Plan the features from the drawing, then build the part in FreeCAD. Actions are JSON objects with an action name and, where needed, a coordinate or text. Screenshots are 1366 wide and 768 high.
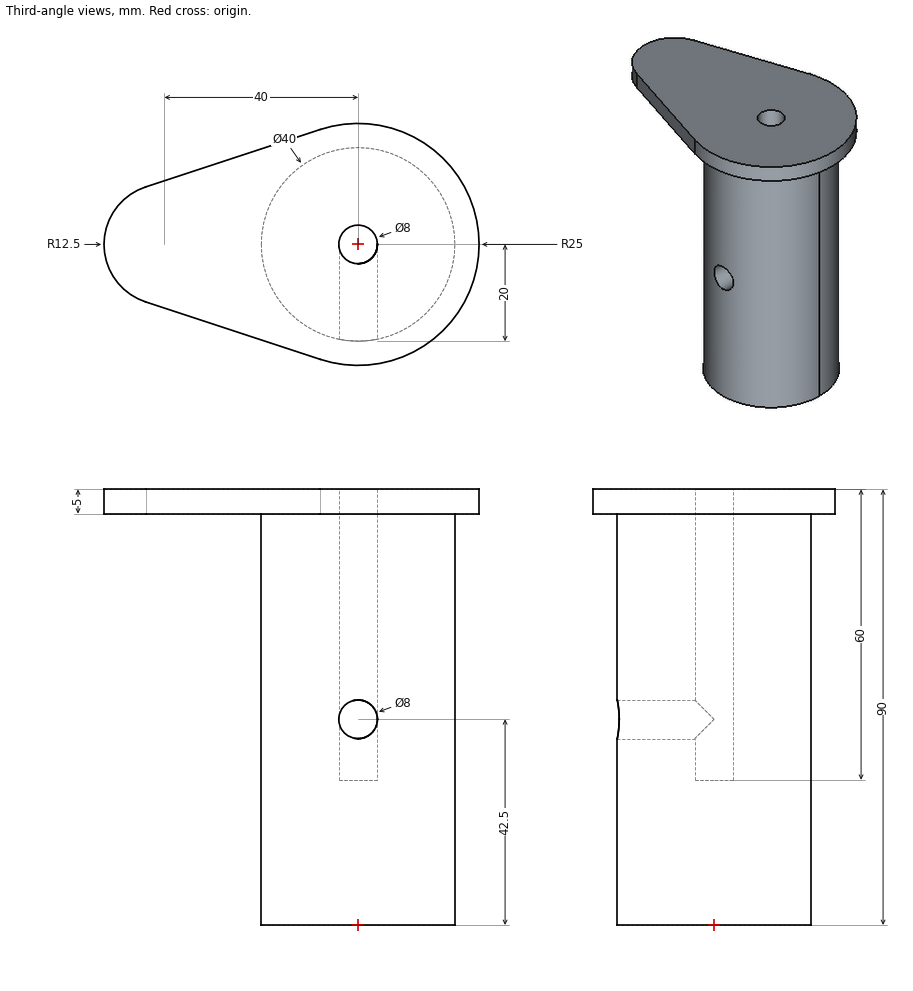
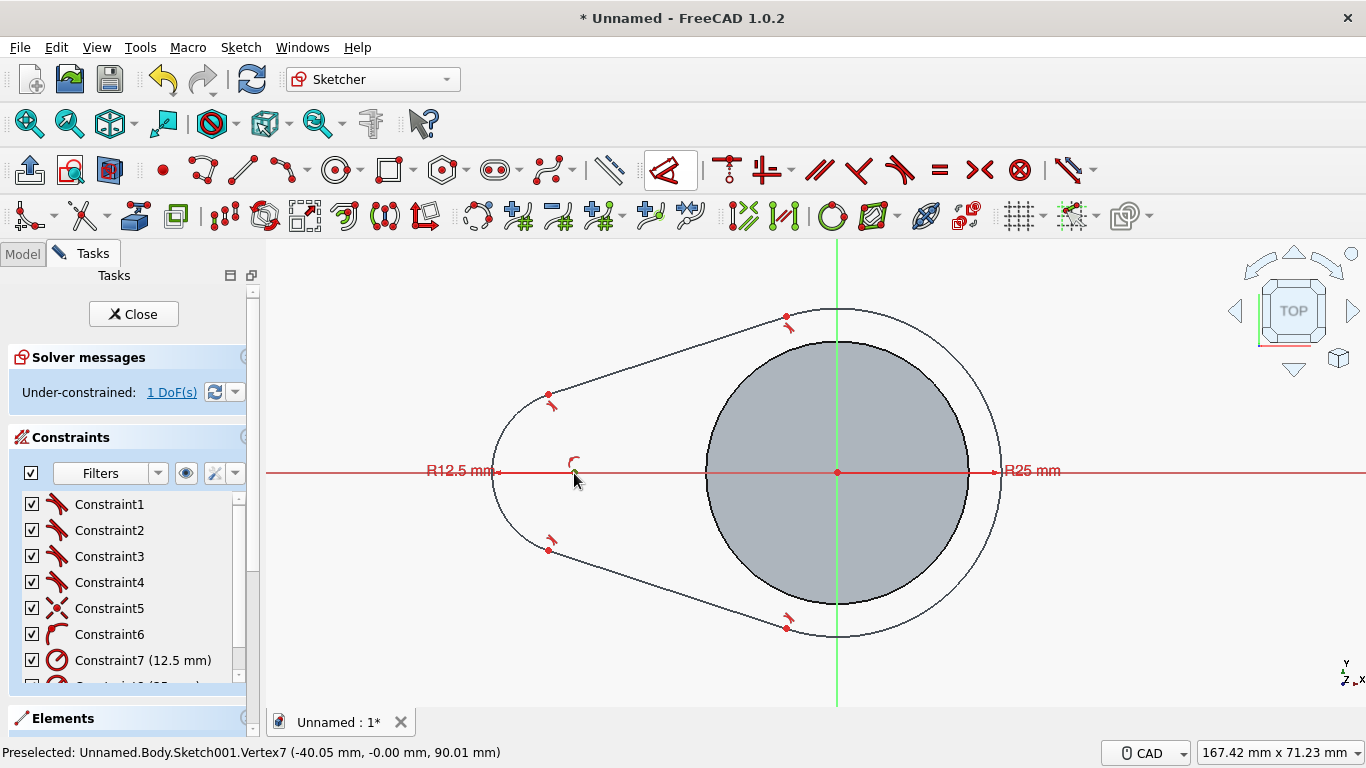
{"action": "key", "text": "l"}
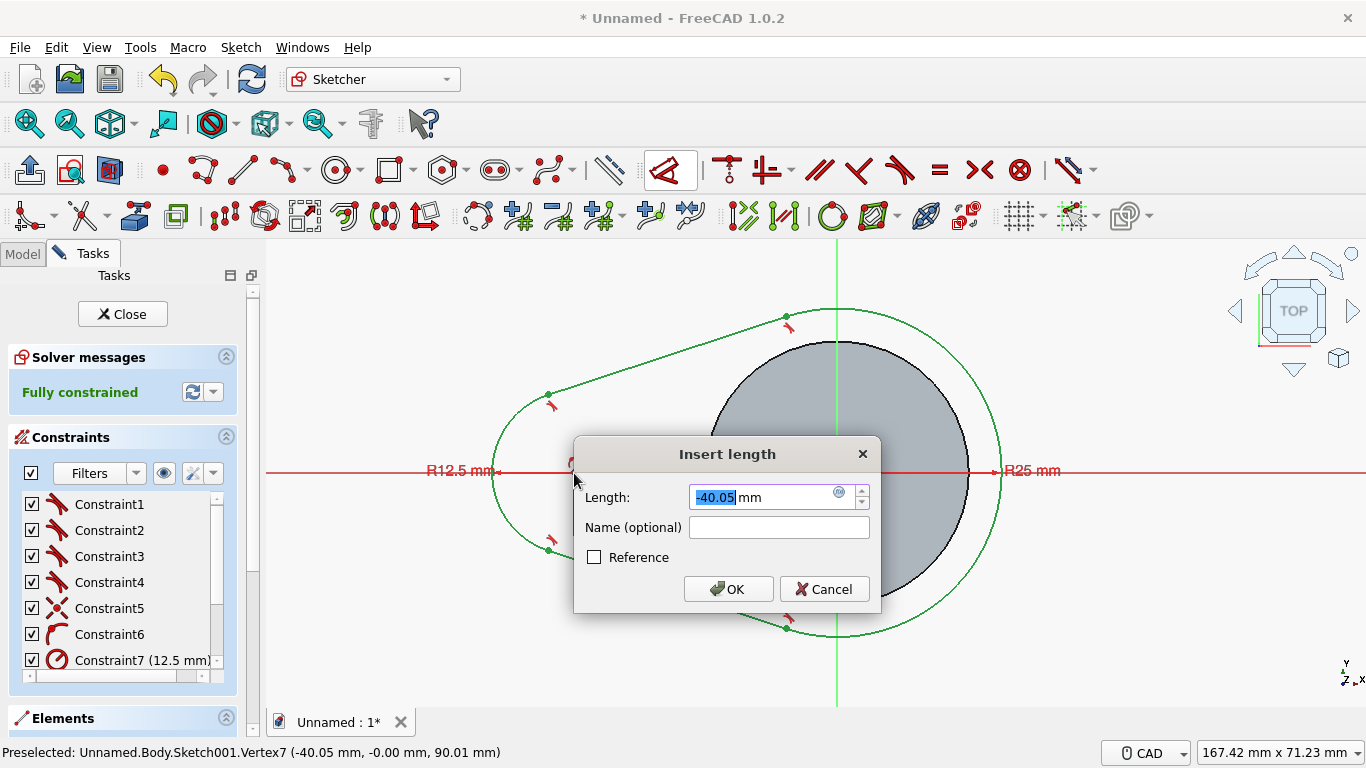
{"action": "type", "text": "-40"}
{"action": "key", "text": "Return"}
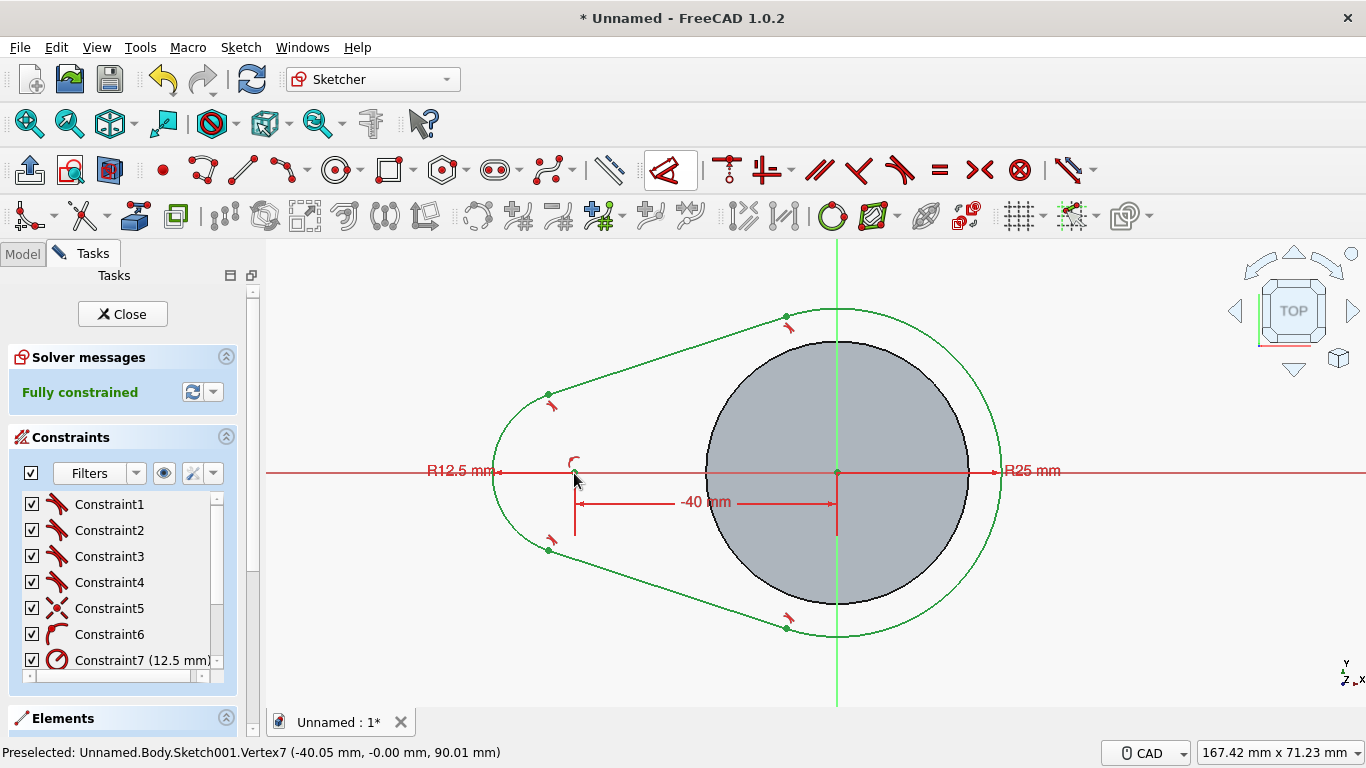
{"action": "left_click", "coordinate": [123, 314]}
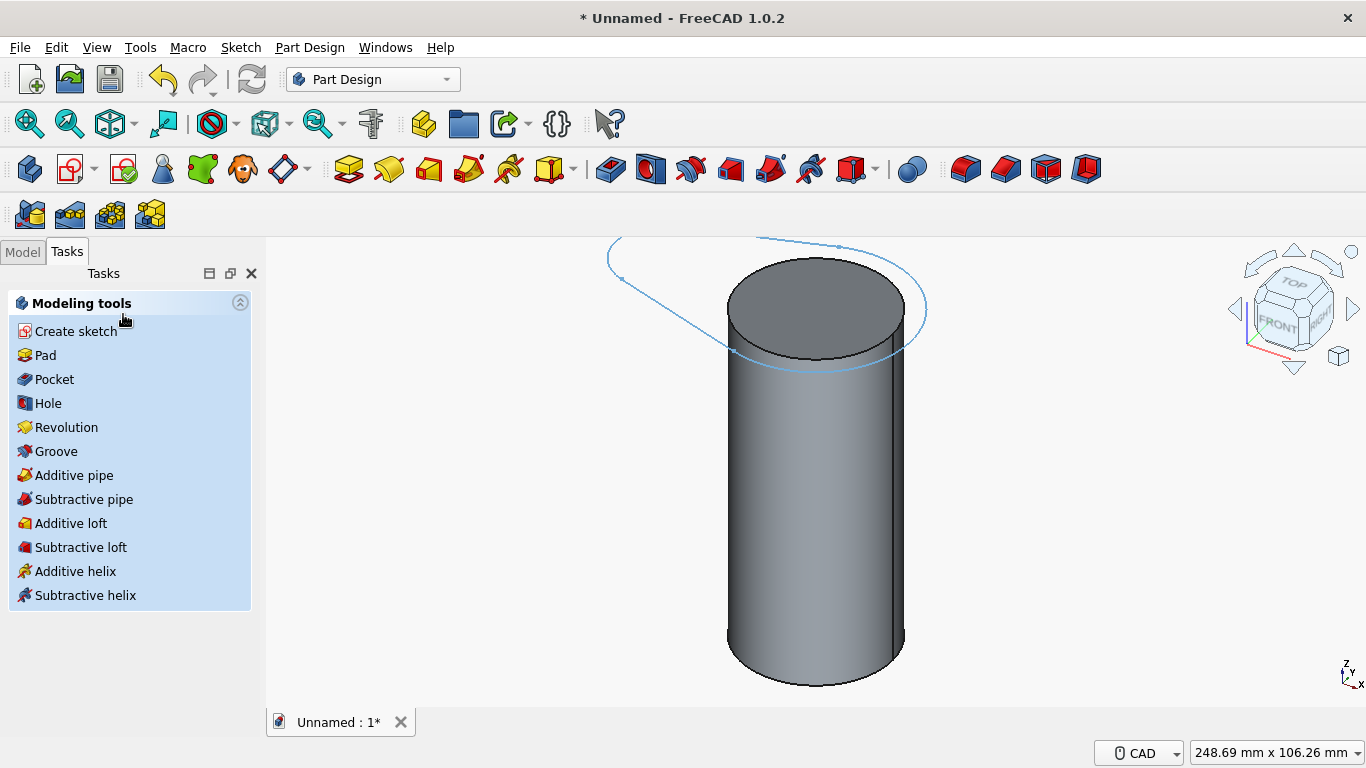
{"action": "left_click", "coordinate": [350, 170]}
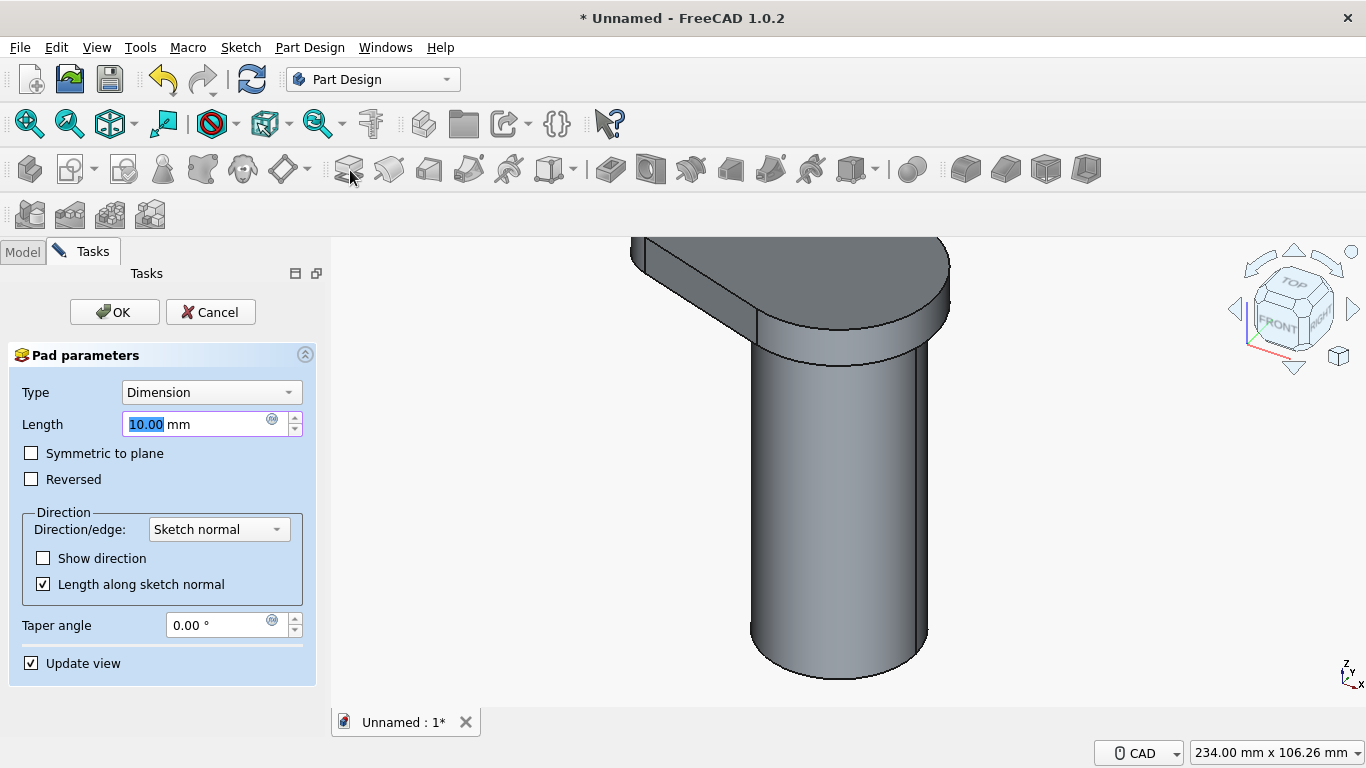
{"action": "type", "text": "5"}
{"action": "key", "text": "Tab"}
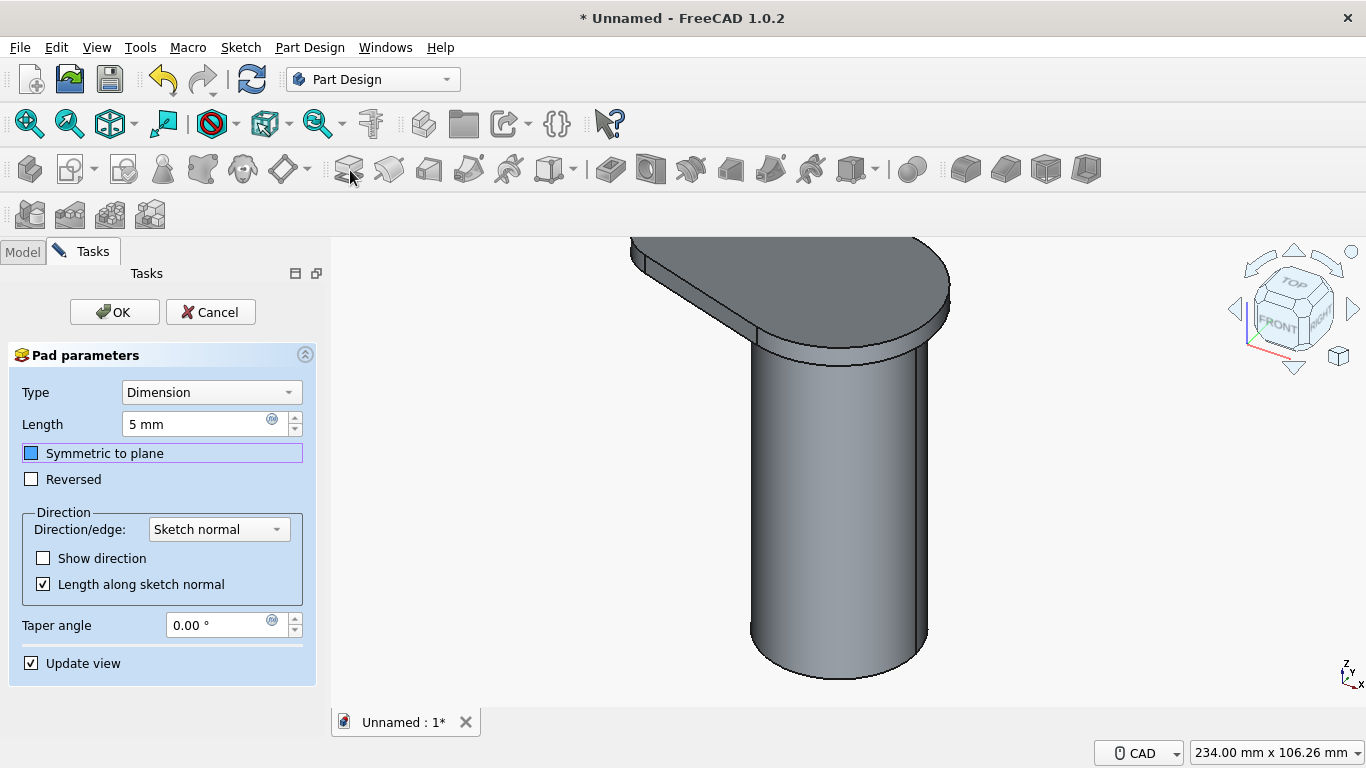
{"action": "left_click", "coordinate": [30, 479]}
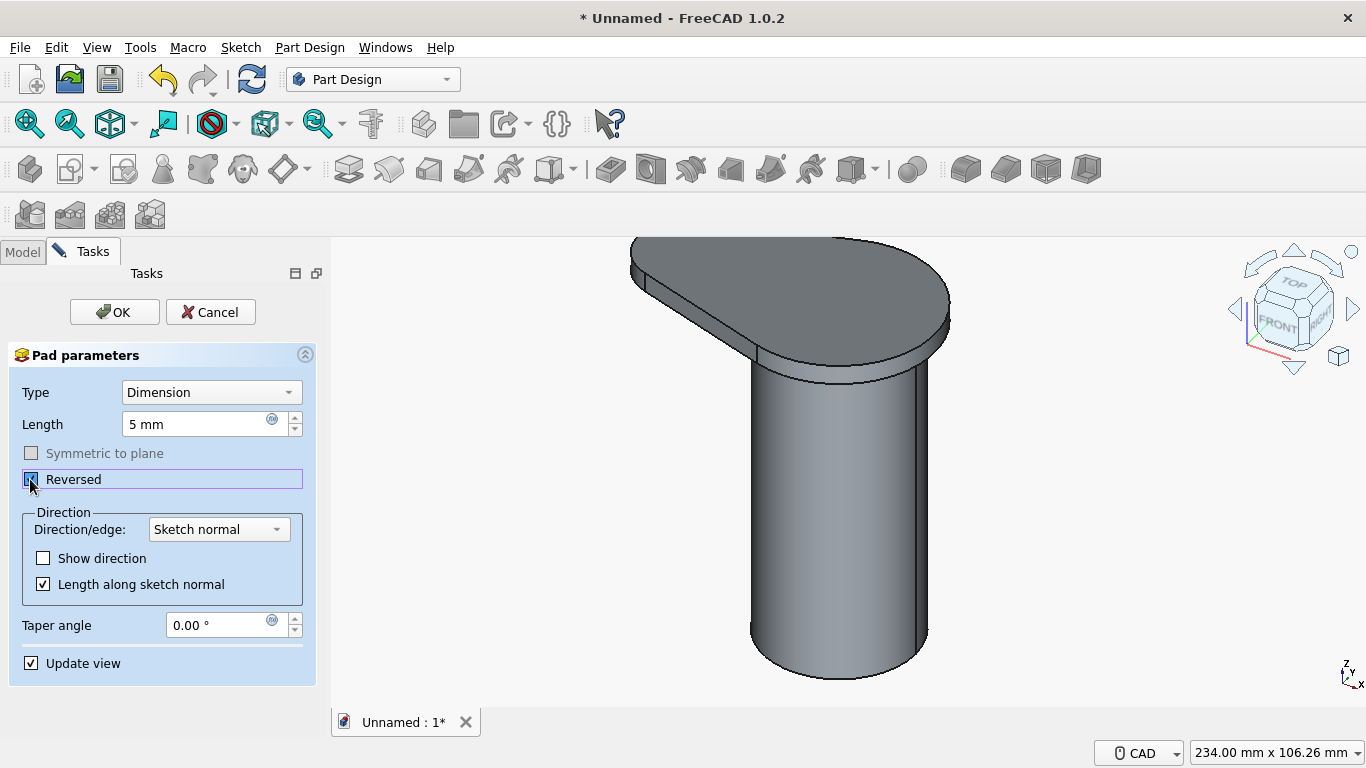
{"action": "left_click", "coordinate": [115, 312]}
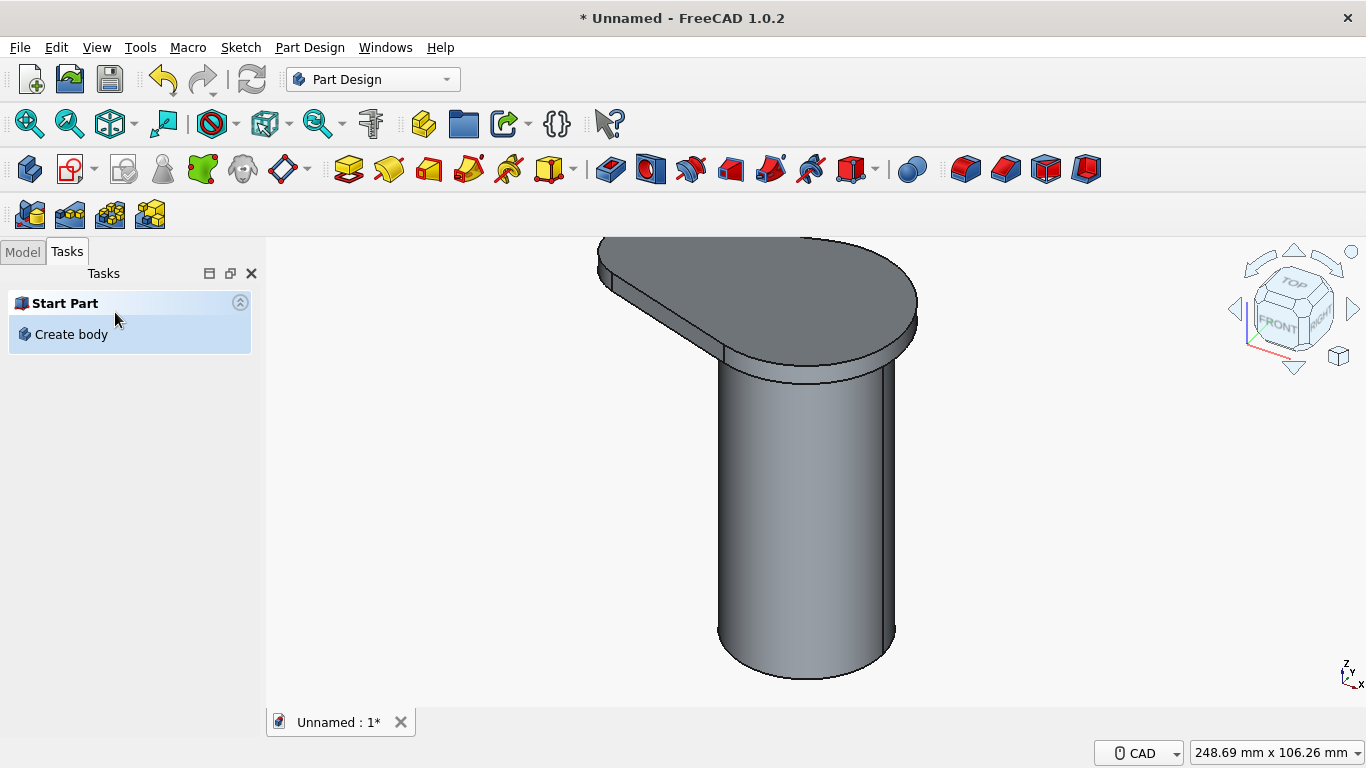
{"action": "key", "text": "v f"}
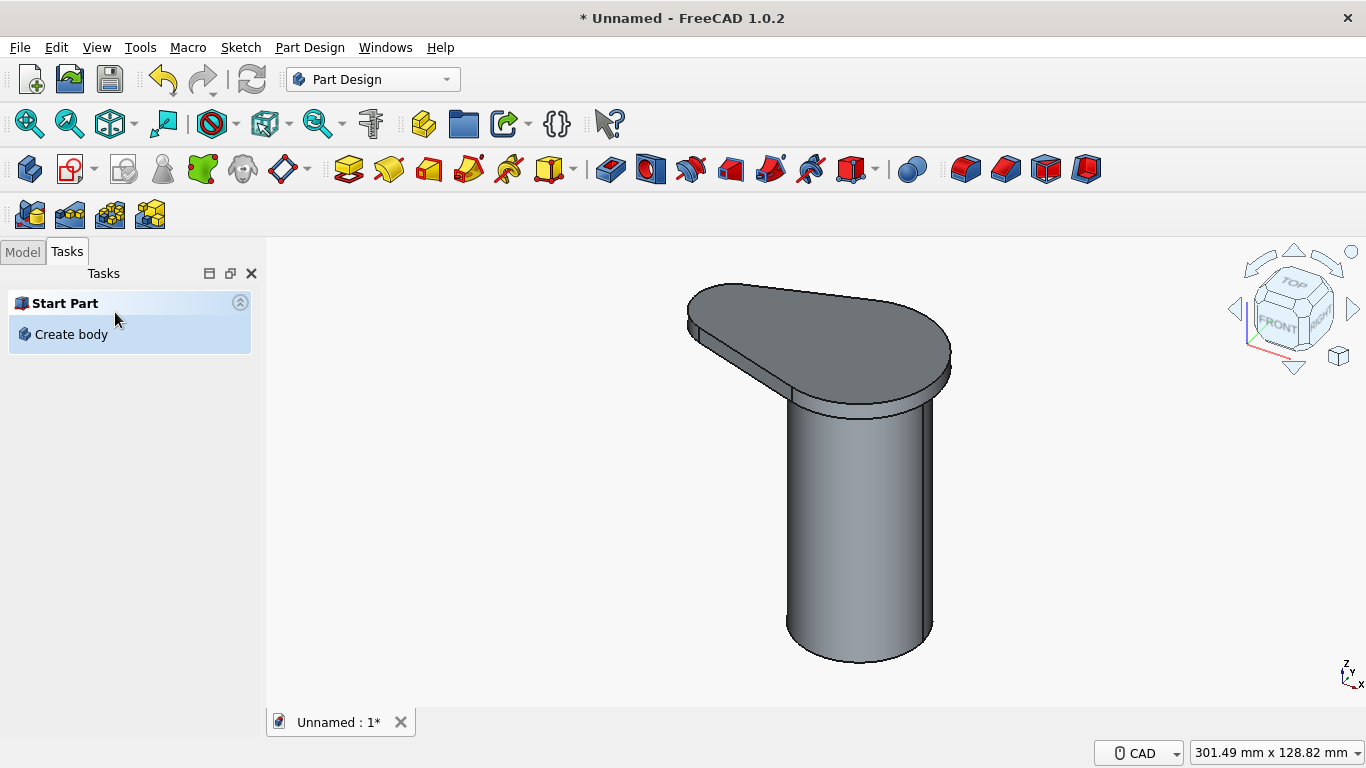
{"action": "left_click", "coordinate": [851, 348]}